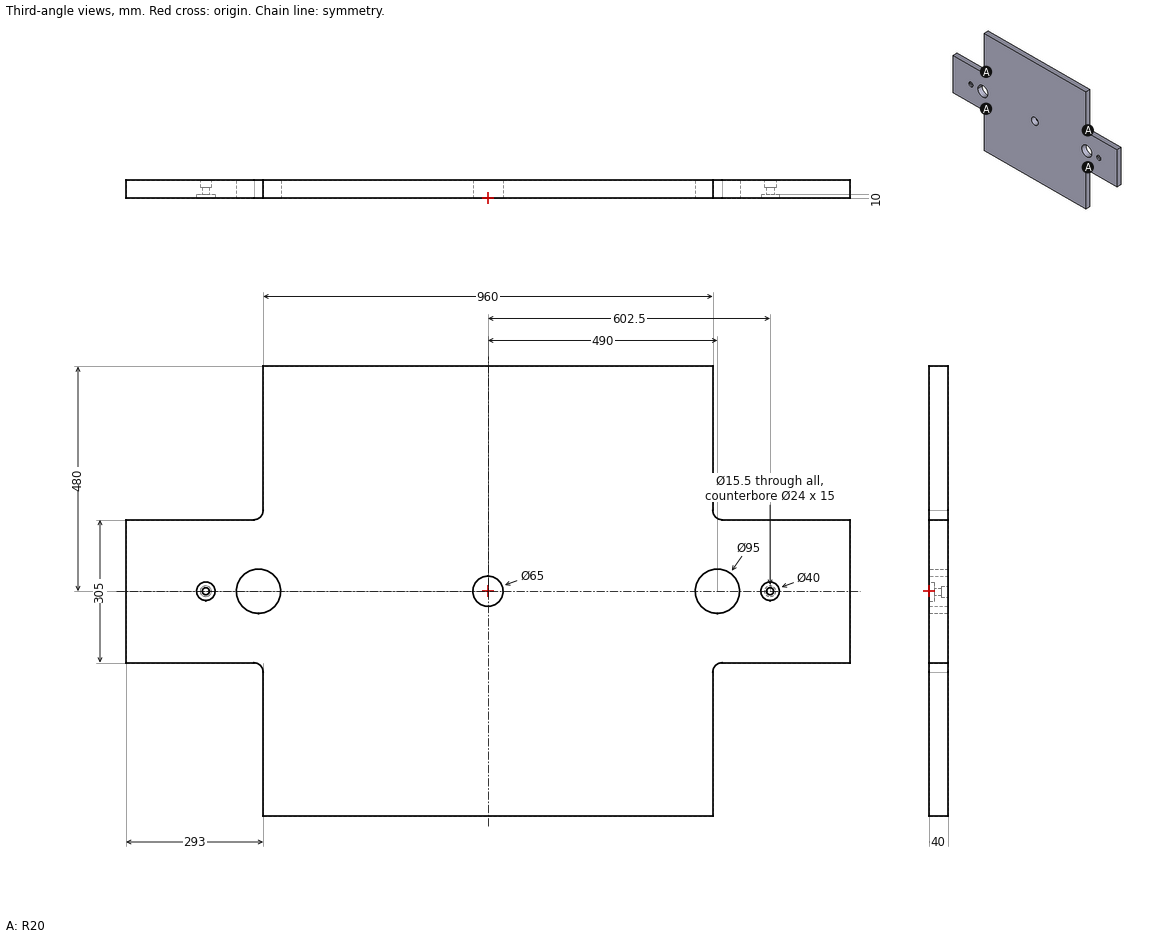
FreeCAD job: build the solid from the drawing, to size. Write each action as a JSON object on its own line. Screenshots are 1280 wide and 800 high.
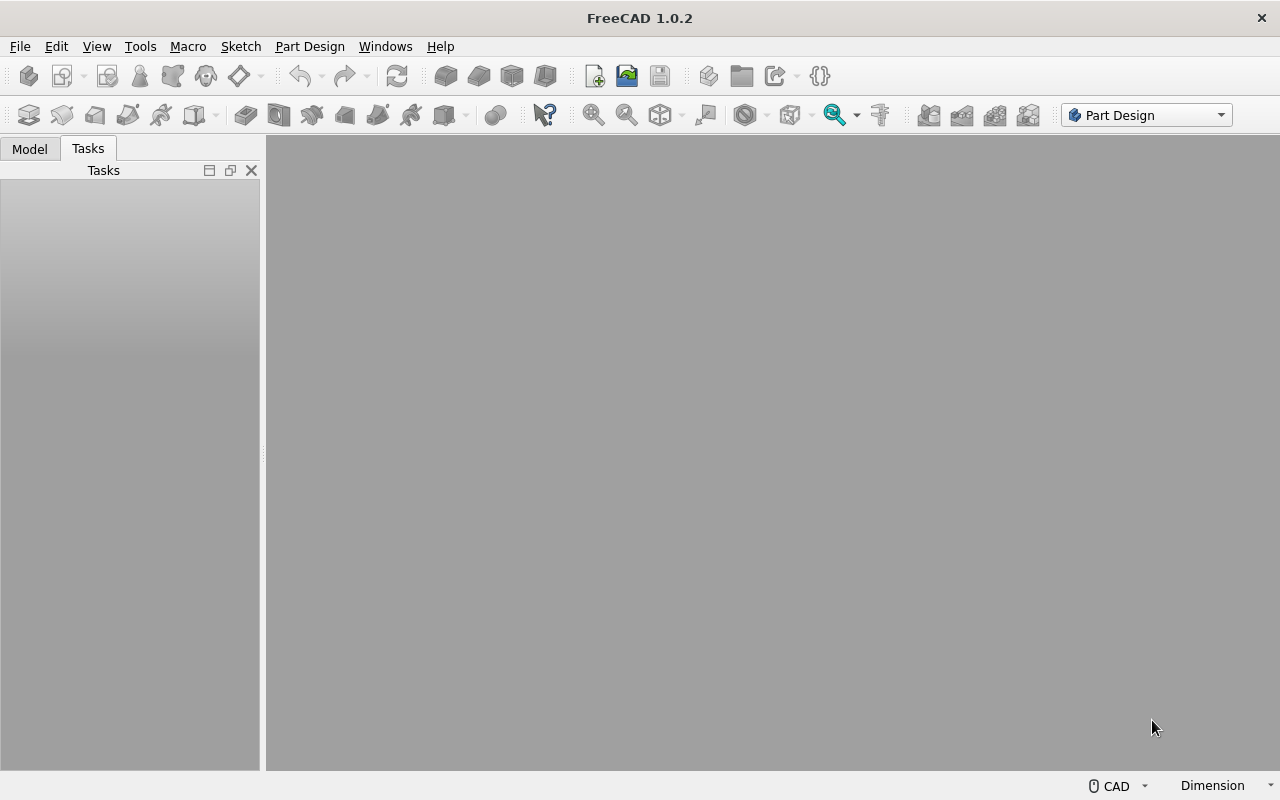
{"action": "key", "text": "ctrl+n"}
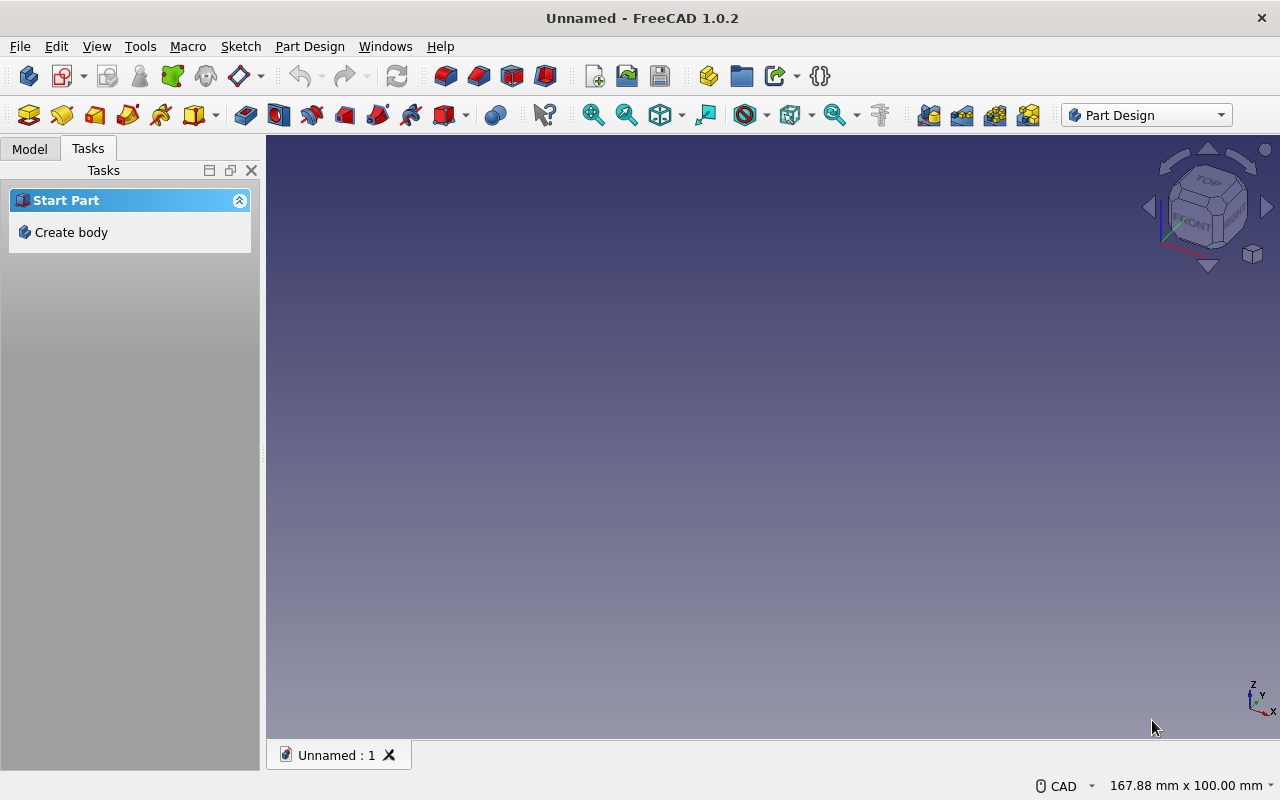
{"action": "left_click", "coordinate": [62, 76]}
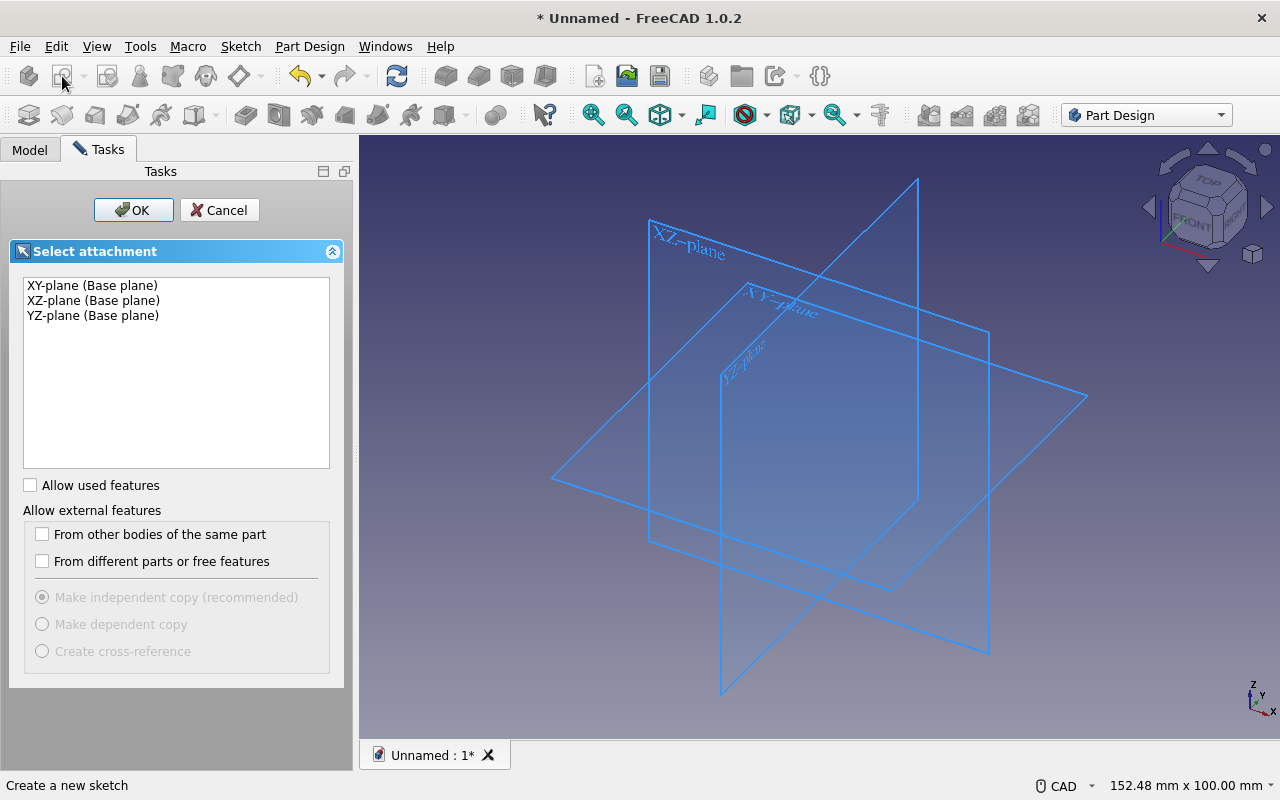
{"action": "left_click", "coordinate": [84, 300]}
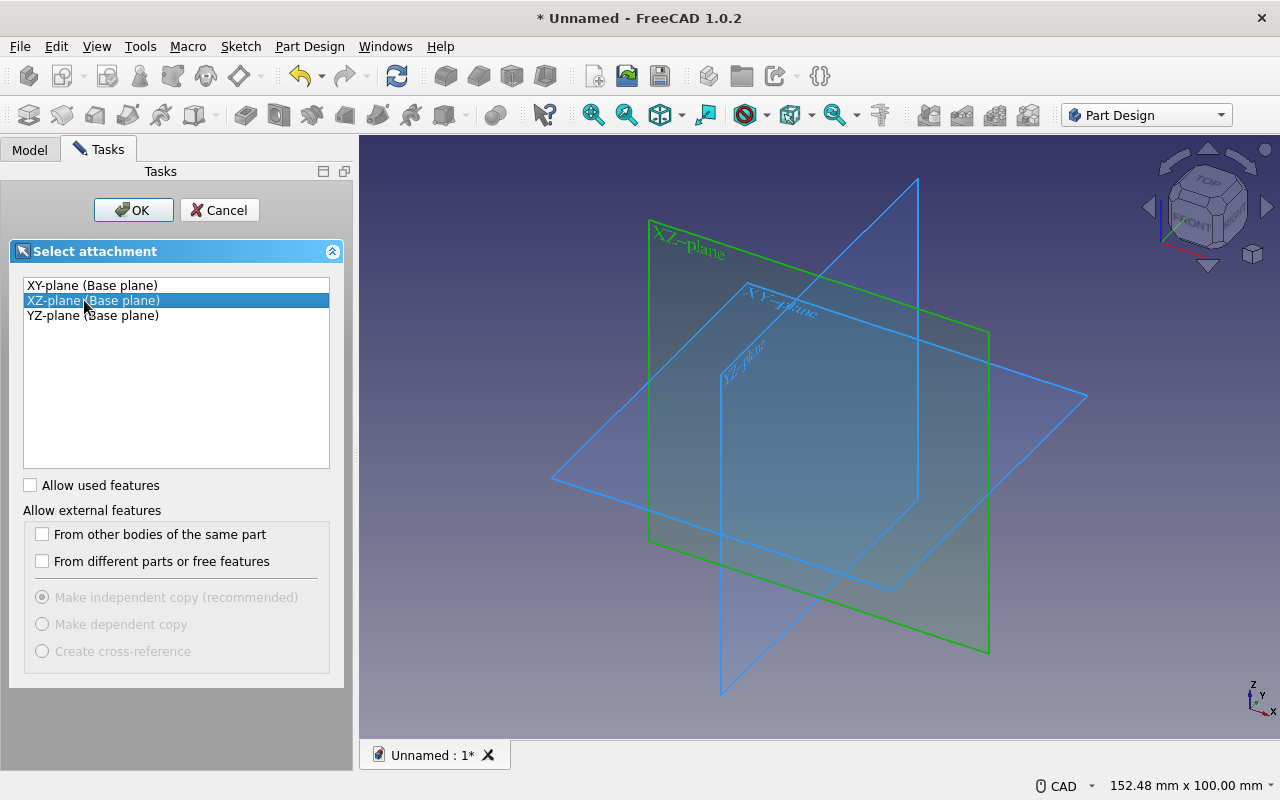
{"action": "left_click", "coordinate": [134, 210]}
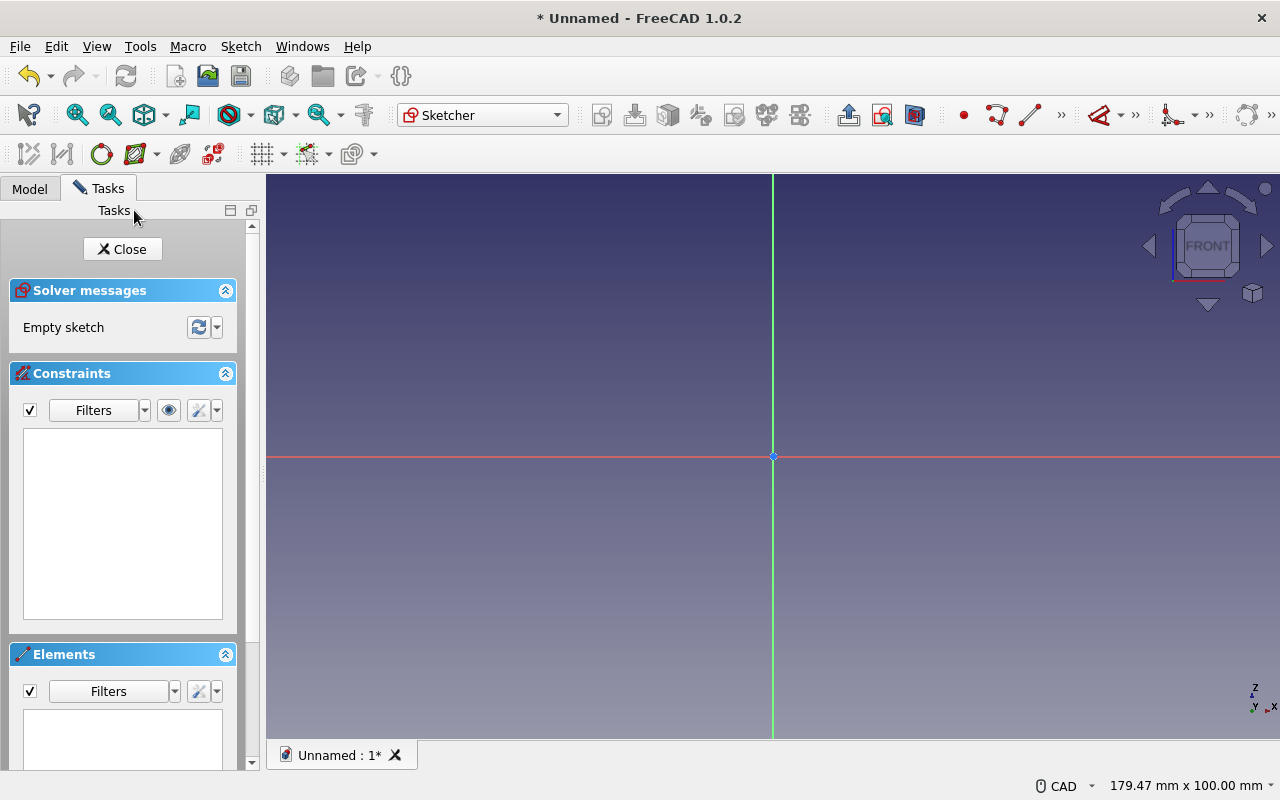
{"action": "scroll", "coordinate": [700, 456], "scroll_direction": "down", "scroll_amount": 14}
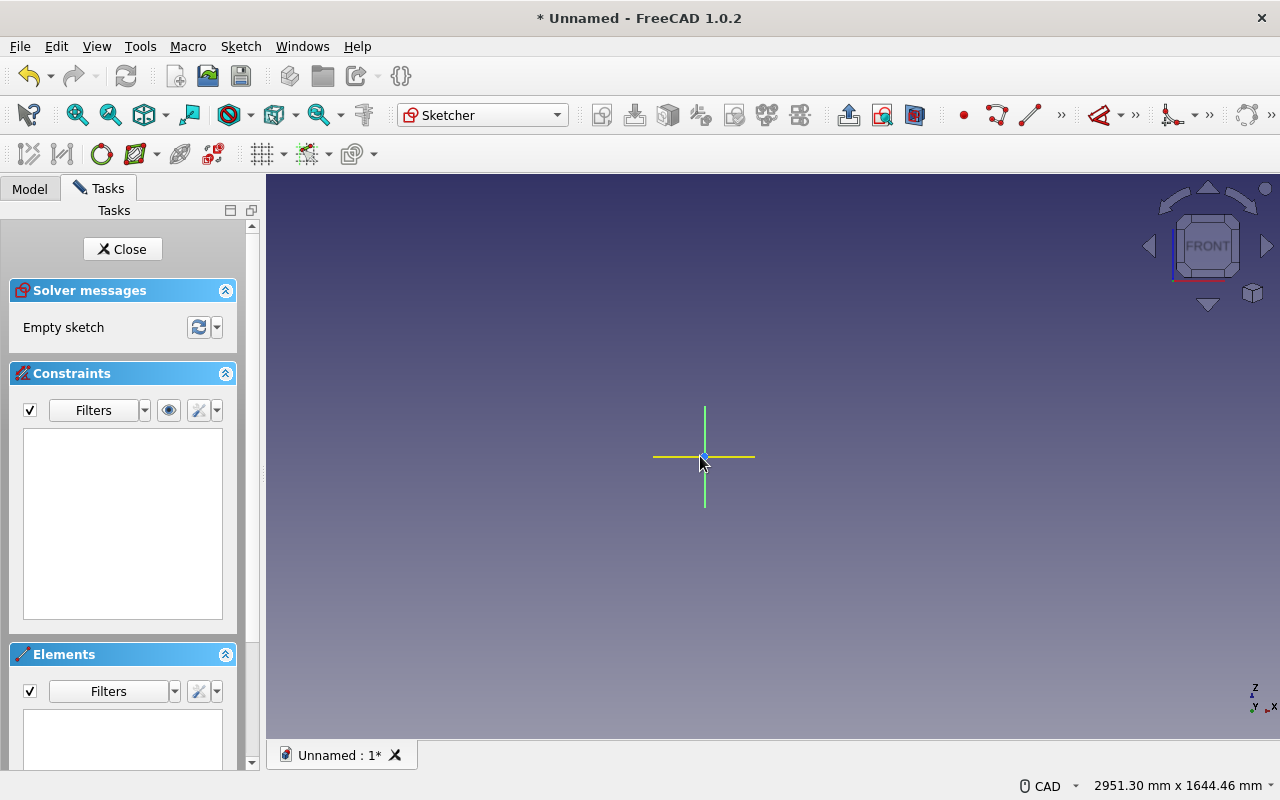
{"action": "key", "text": "g m"}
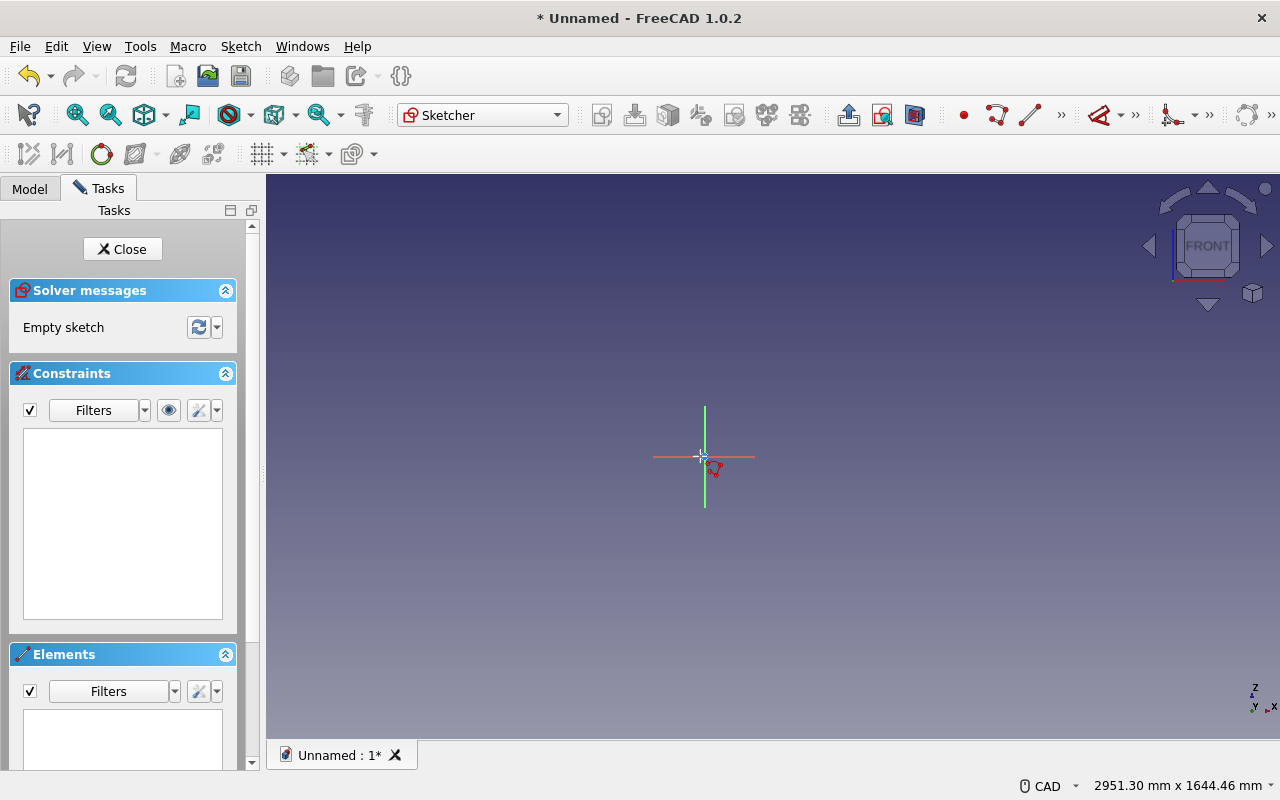
{"action": "left_click", "coordinate": [540, 509]}
{"action": "left_click", "coordinate": [439, 509]}
{"action": "left_click", "coordinate": [439, 404]}
{"action": "left_click", "coordinate": [540, 404]}
{"action": "left_click", "coordinate": [540, 292]}
{"action": "left_click", "coordinate": [870, 292]}
{"action": "left_click", "coordinate": [870, 404]}
{"action": "left_click", "coordinate": [970, 404]}
{"action": "left_click", "coordinate": [970, 509]}
{"action": "left_click", "coordinate": [870, 509]}
{"action": "left_click", "coordinate": [870, 621]}
{"action": "left_click", "coordinate": [540, 621]}
{"action": "left_click", "coordinate": [540, 510]}
{"action": "key", "text": "Escape"}
{"action": "key", "text": "Escape"}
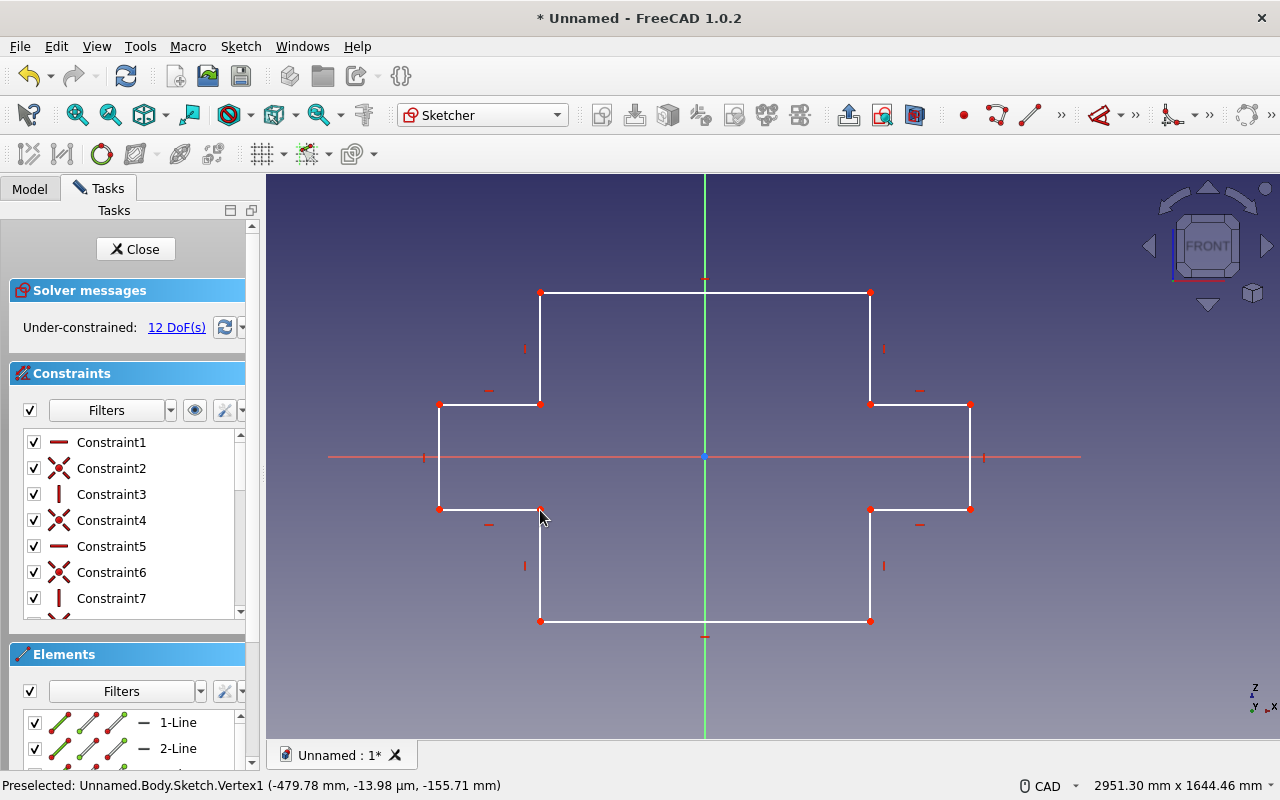
{"action": "left_click", "coordinate": [540, 510]}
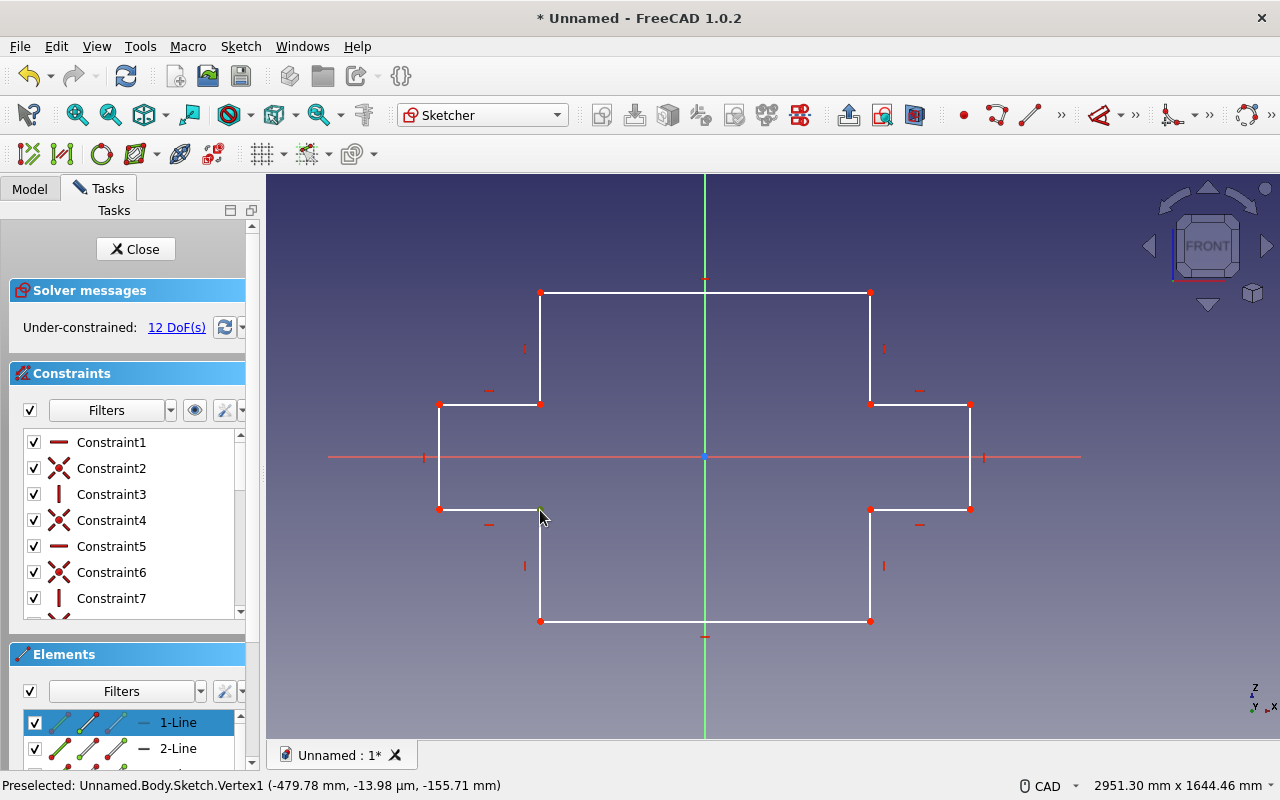
{"action": "left_click", "coordinate": [540, 405]}